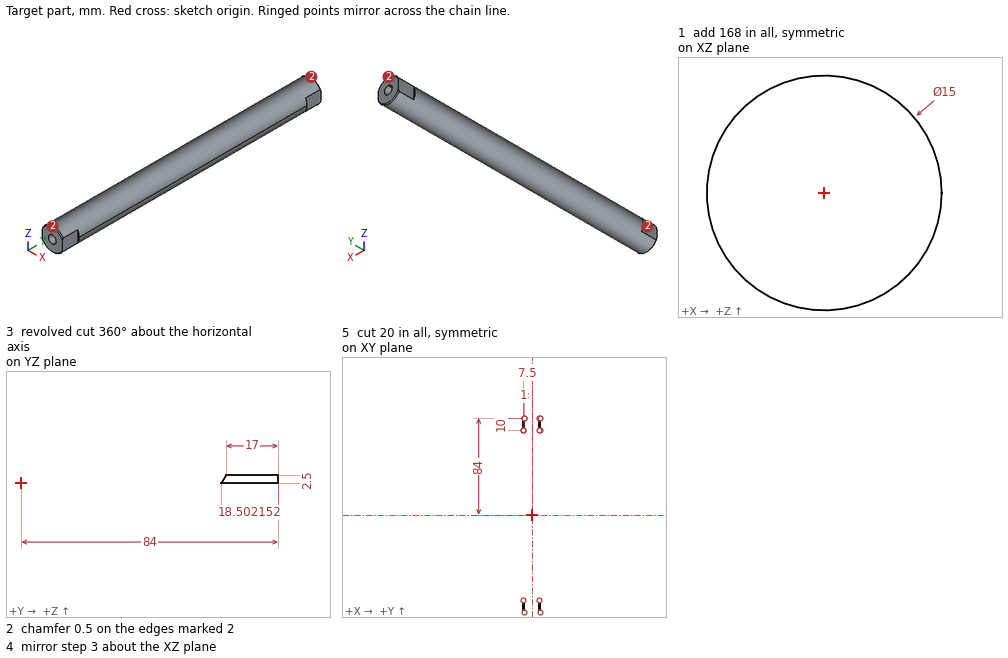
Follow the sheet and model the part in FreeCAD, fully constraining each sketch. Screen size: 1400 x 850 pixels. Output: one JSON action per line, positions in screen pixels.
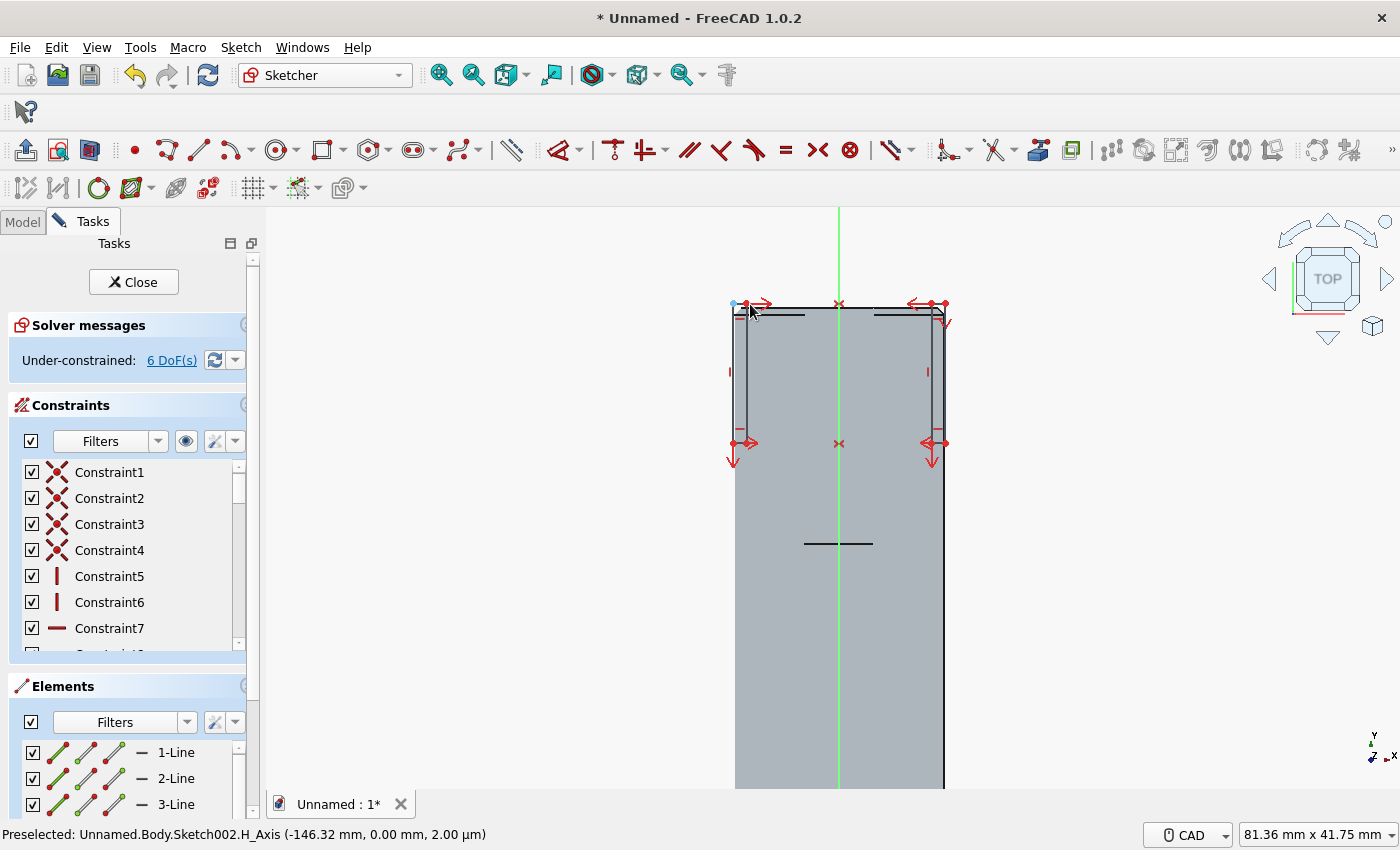
{"action": "left_click", "coordinate": [747, 304]}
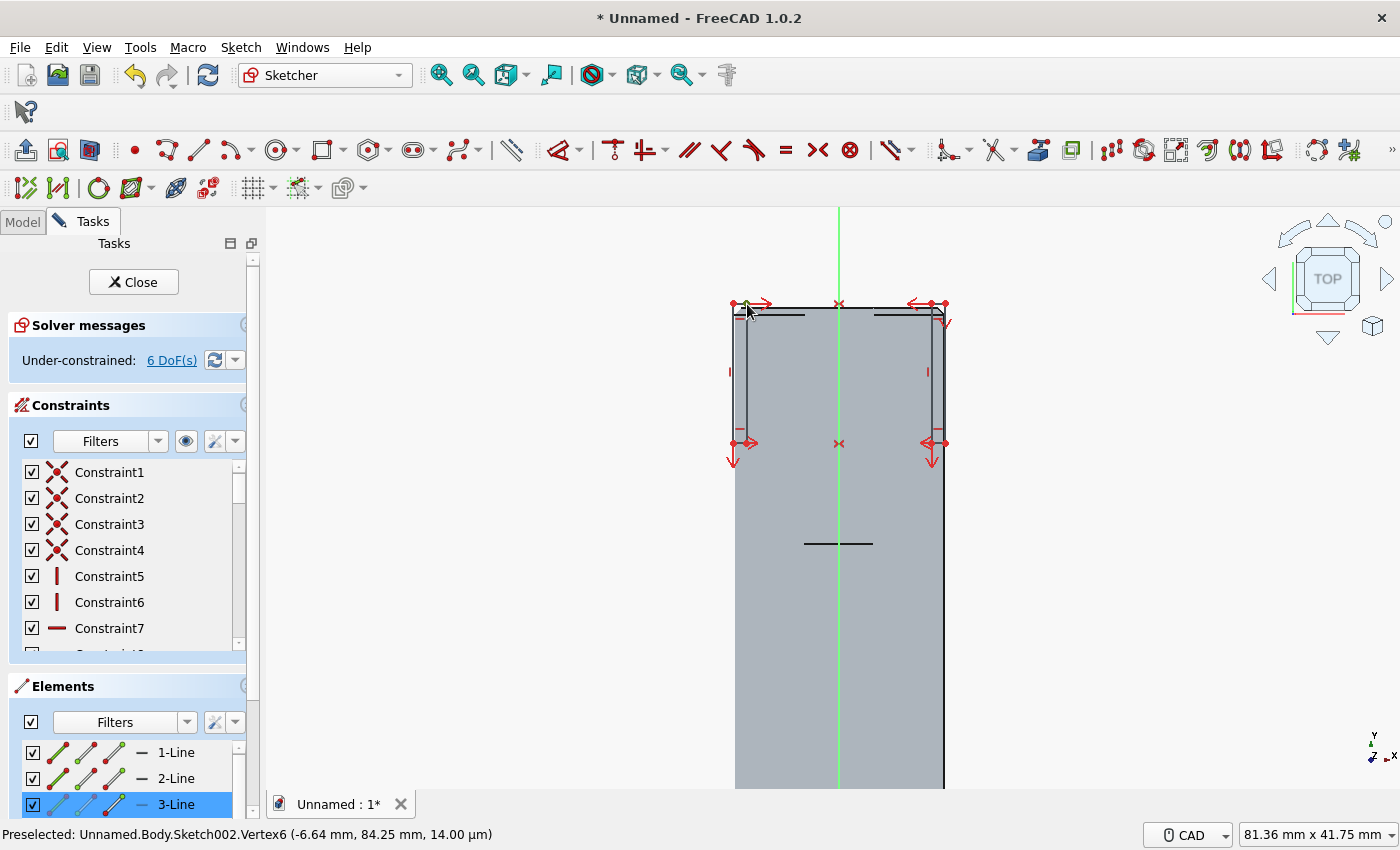
{"action": "scroll", "coordinate": [750, 304], "scroll_direction": "down", "scroll_amount": 9}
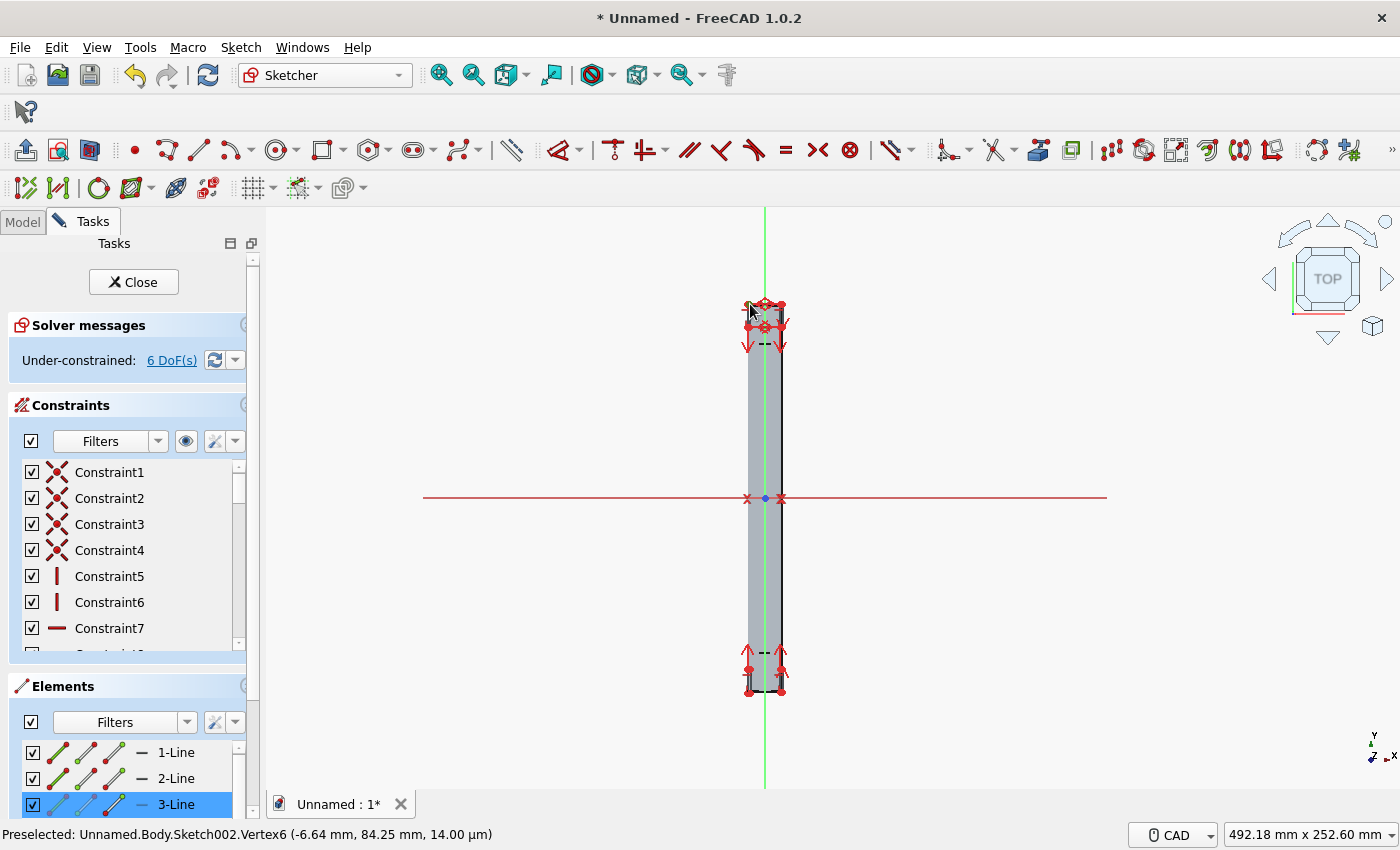
{"action": "scroll", "coordinate": [751, 693], "scroll_direction": "up", "scroll_amount": 8}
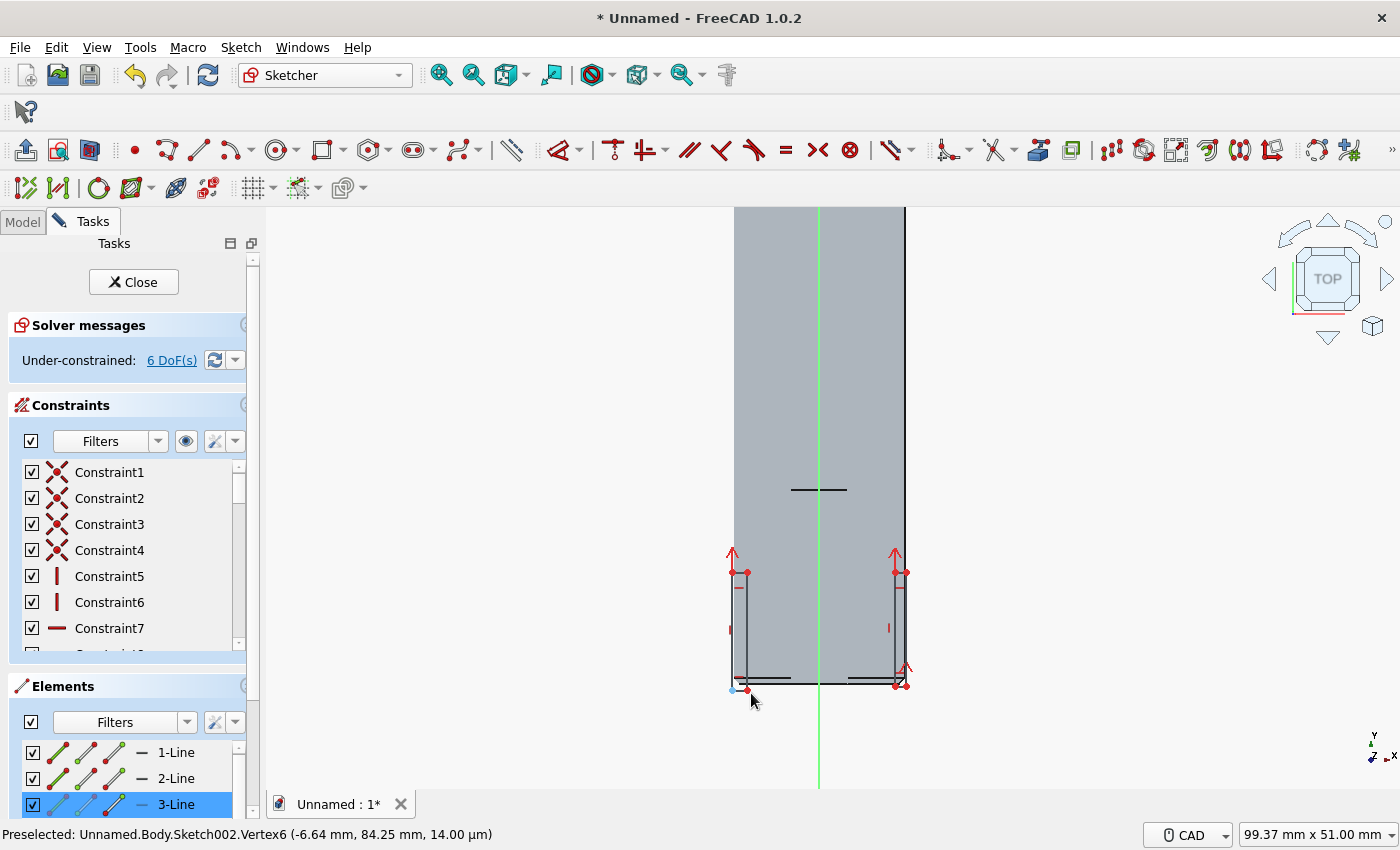
{"action": "left_click", "coordinate": [747, 691]}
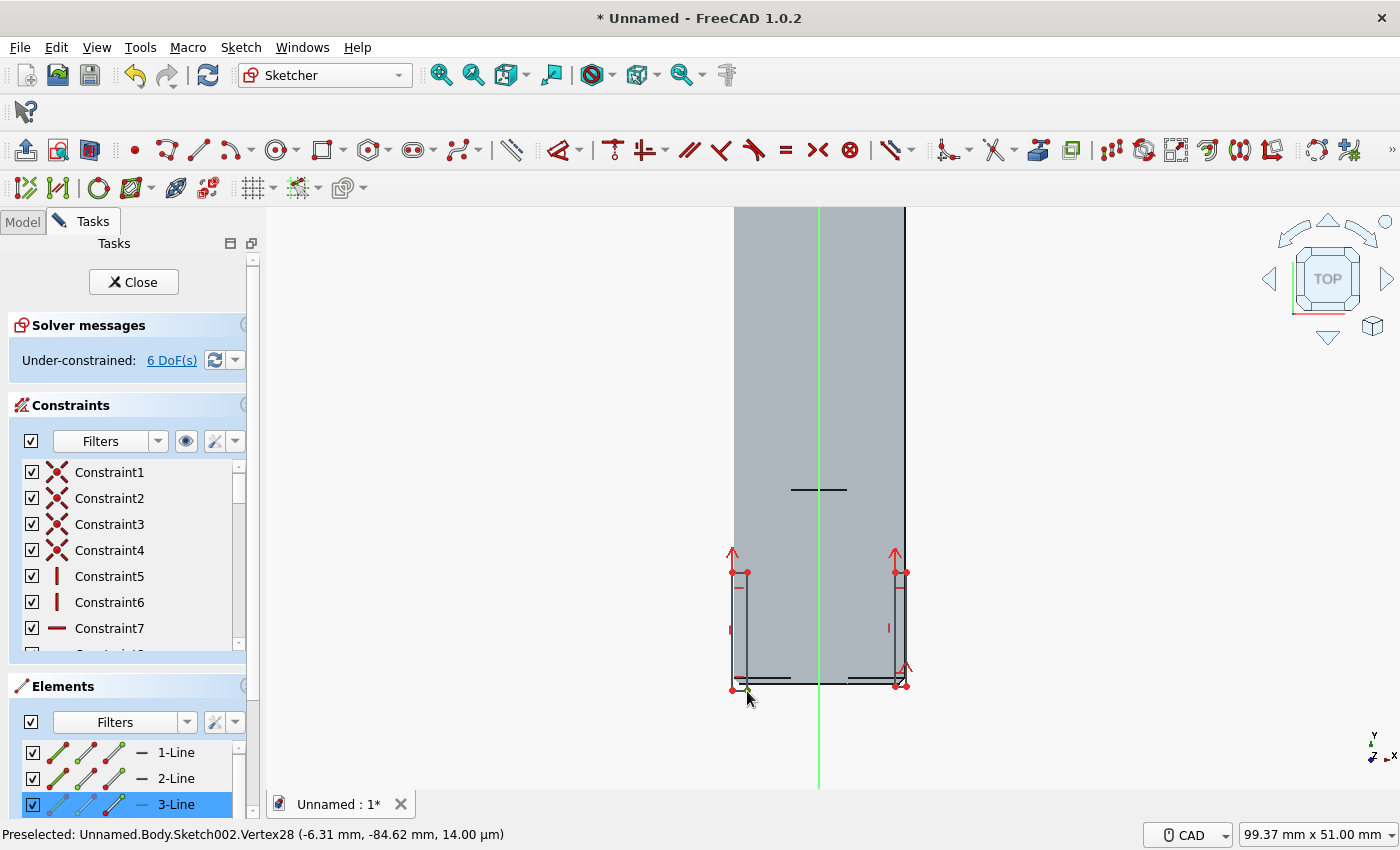
{"action": "scroll", "coordinate": [751, 694], "scroll_direction": "down", "scroll_amount": 8}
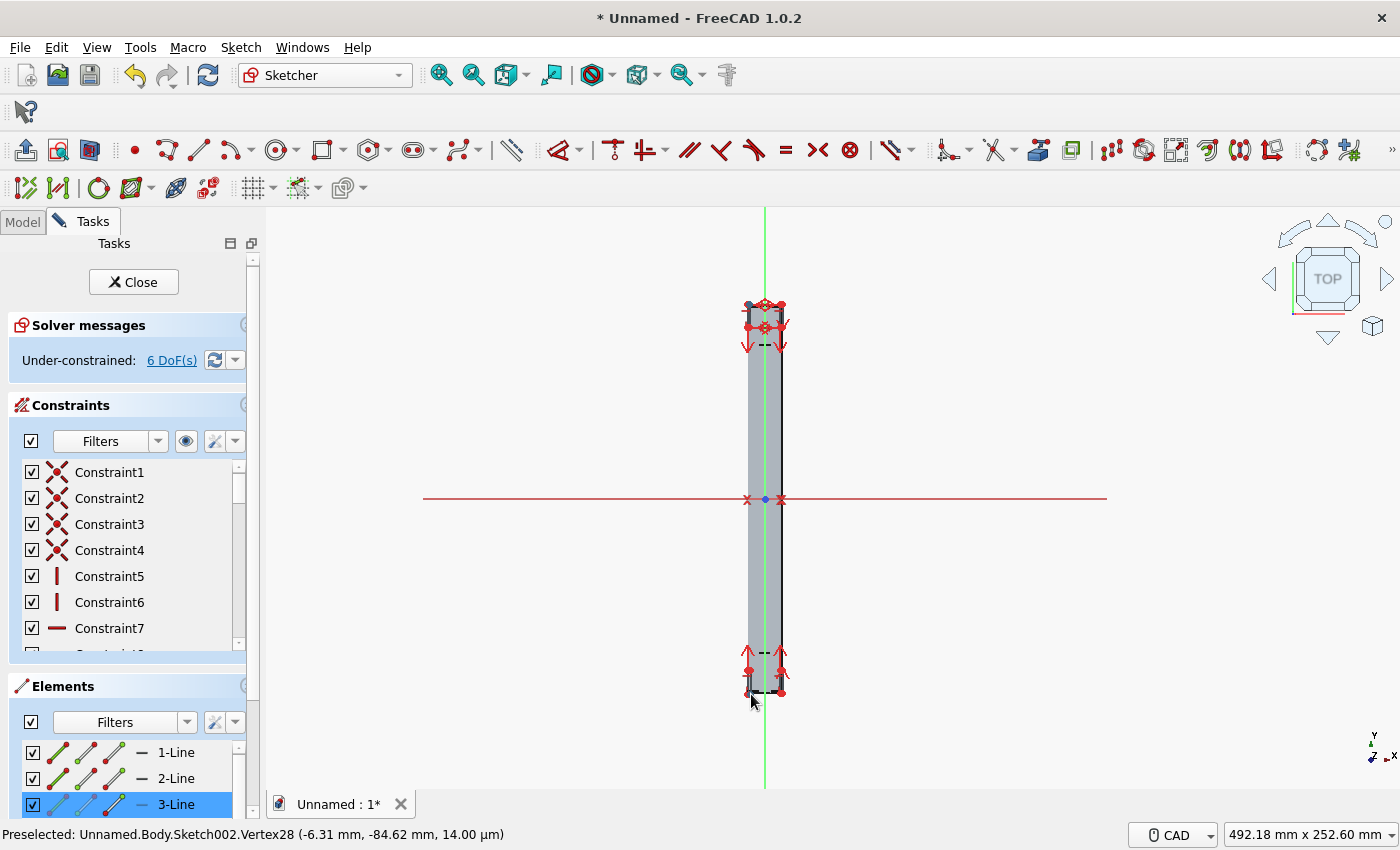
{"action": "left_click", "coordinate": [428, 499]}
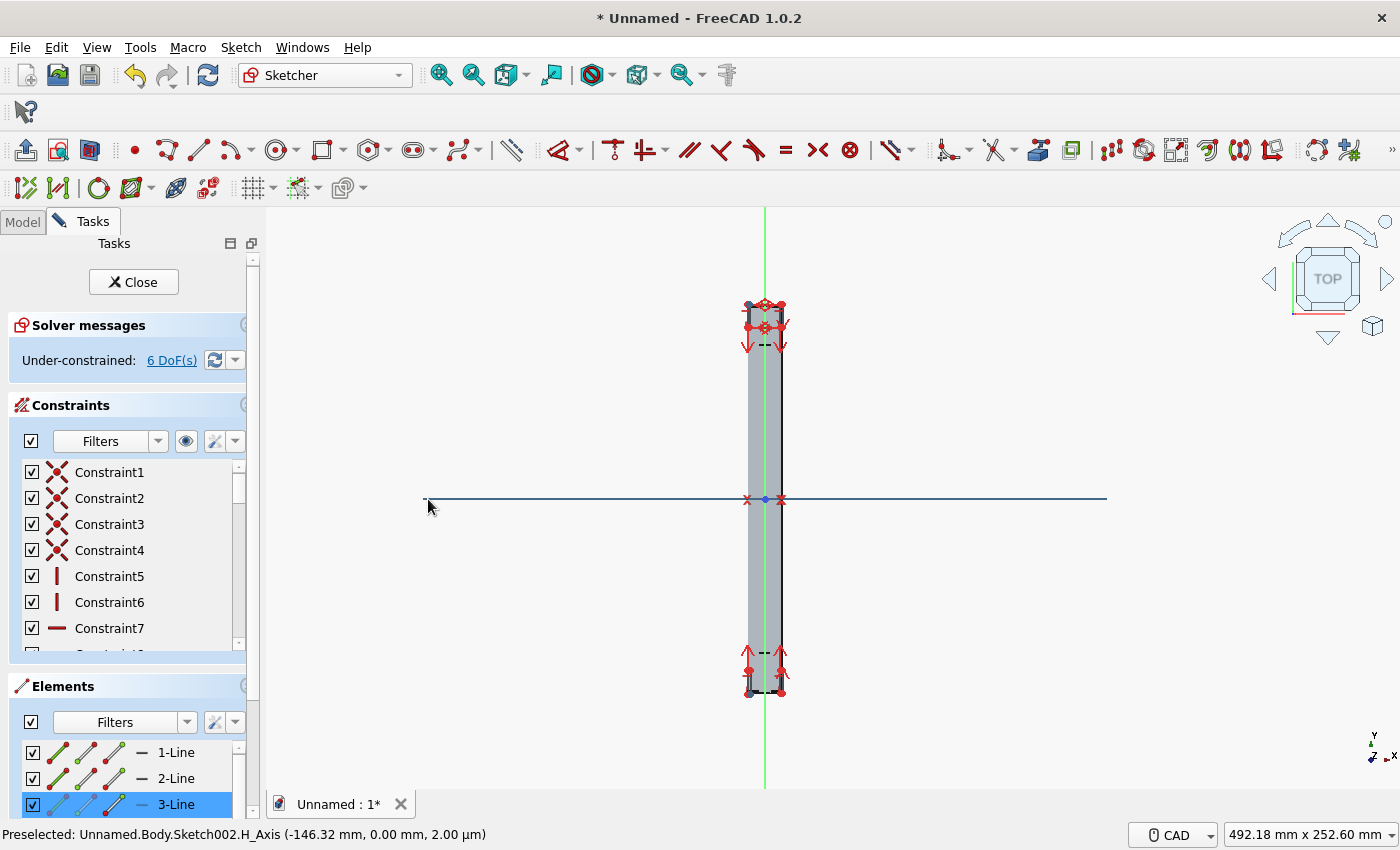
{"action": "left_click", "coordinate": [818, 150]}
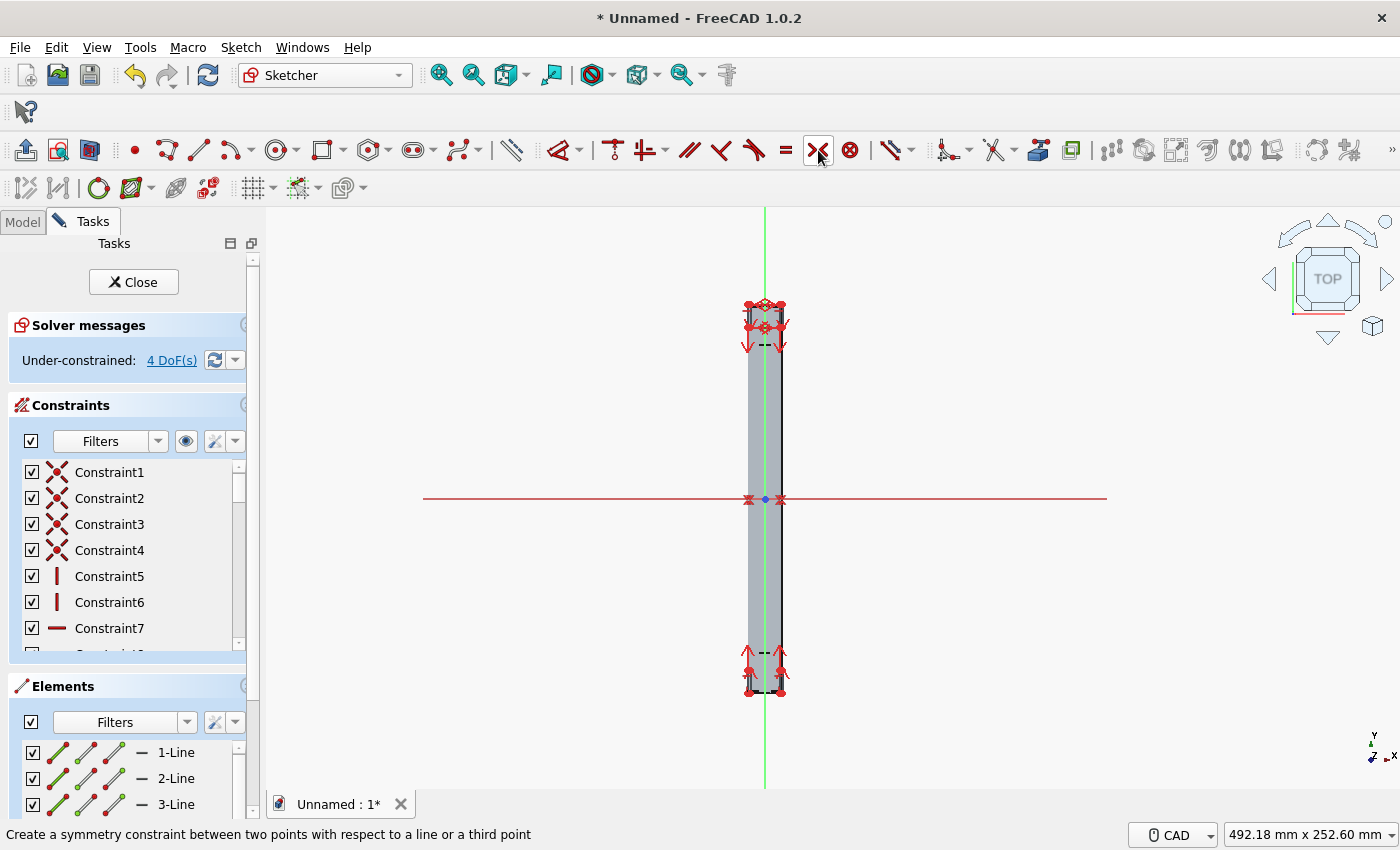
{"action": "left_click", "coordinate": [558, 150]}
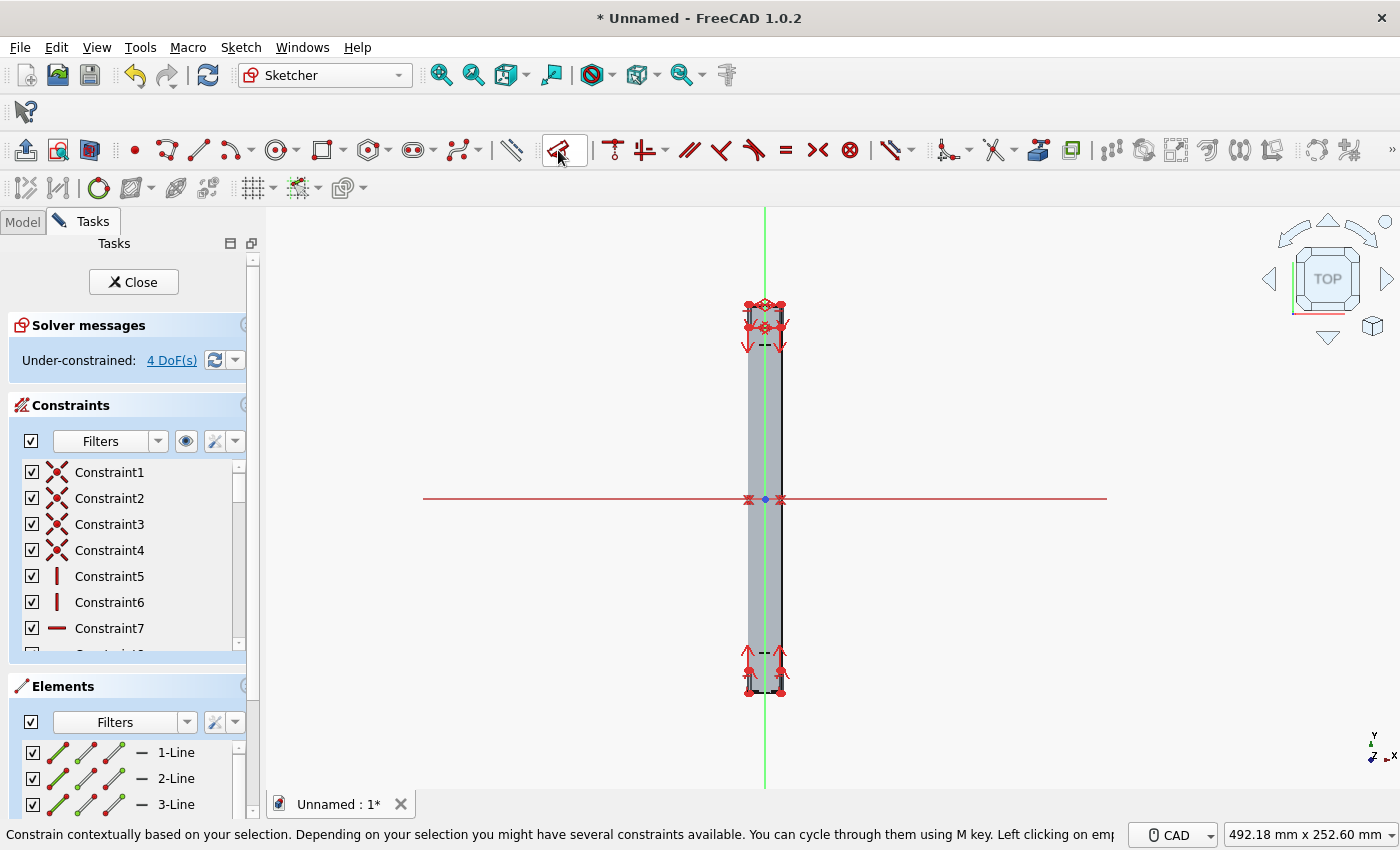
{"action": "scroll", "coordinate": [749, 328], "scroll_direction": "up", "scroll_amount": 15}